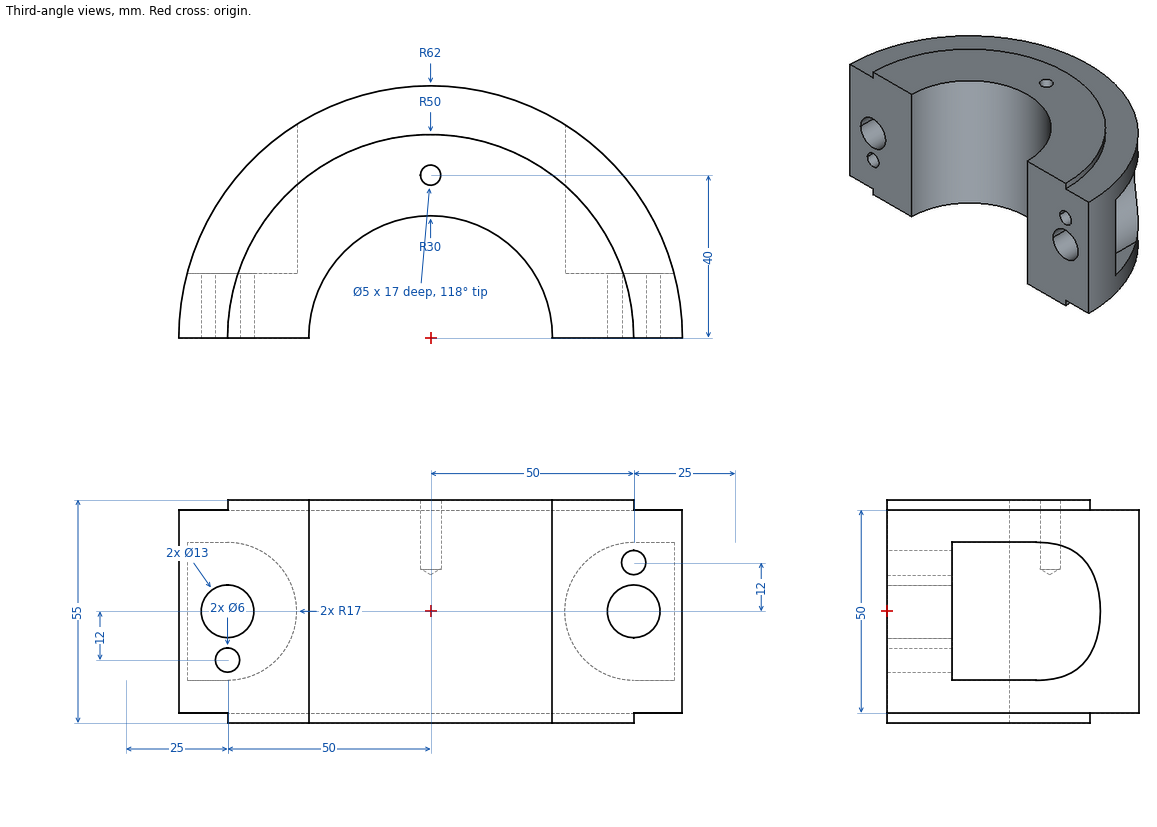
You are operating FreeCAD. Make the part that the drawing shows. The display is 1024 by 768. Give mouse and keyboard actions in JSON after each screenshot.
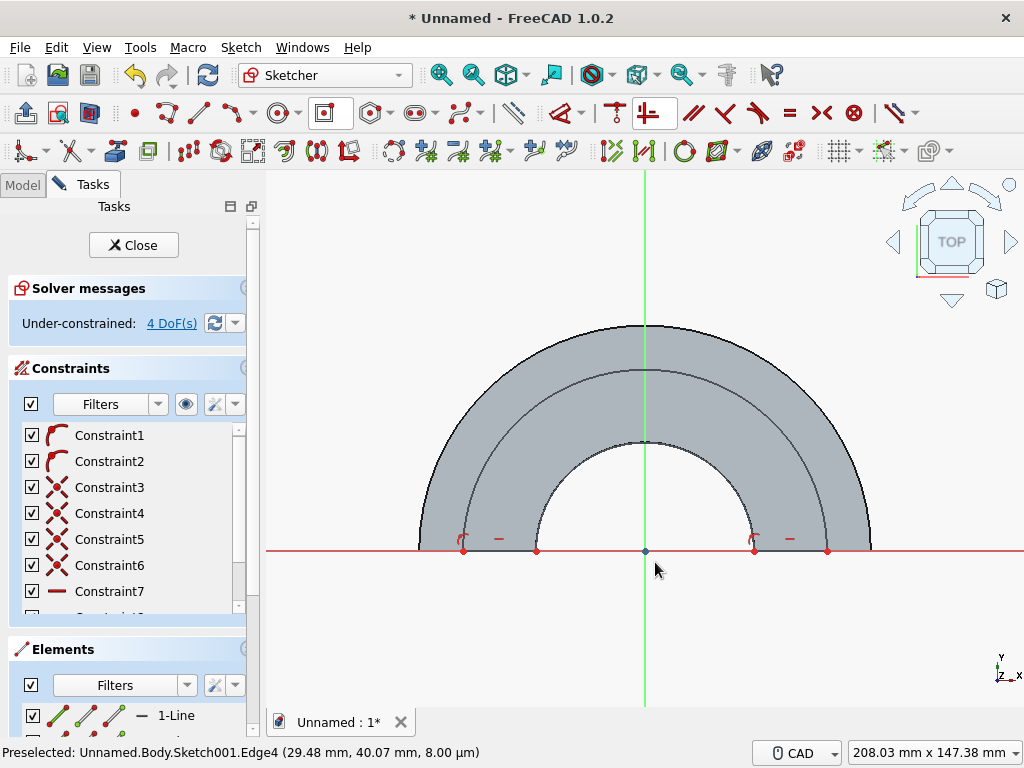
{"action": "left_click", "coordinate": [616, 114]}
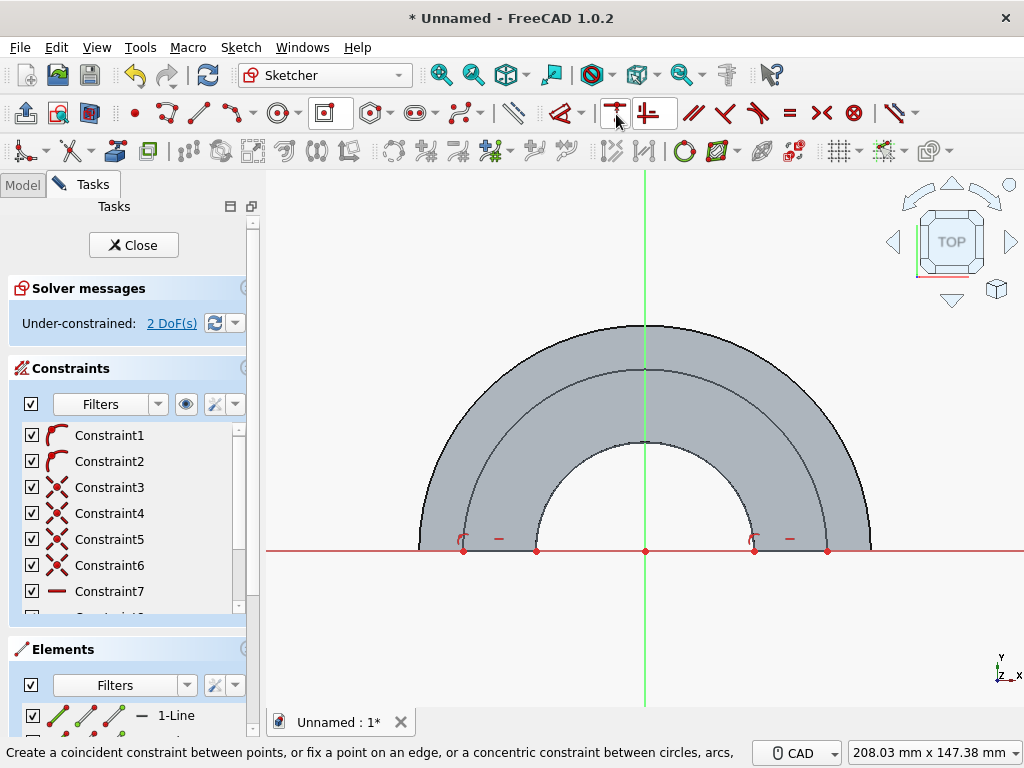
{"action": "left_click", "coordinate": [560, 114]}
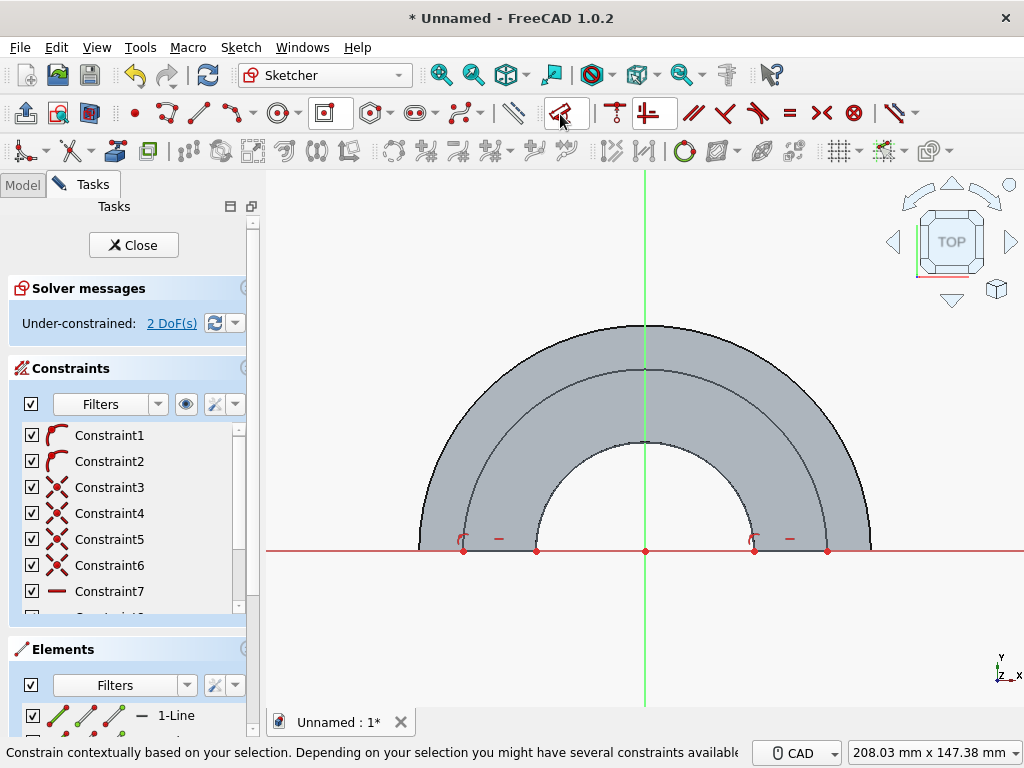
{"action": "left_click", "coordinate": [709, 463]}
{"action": "left_click", "coordinate": [728, 437]}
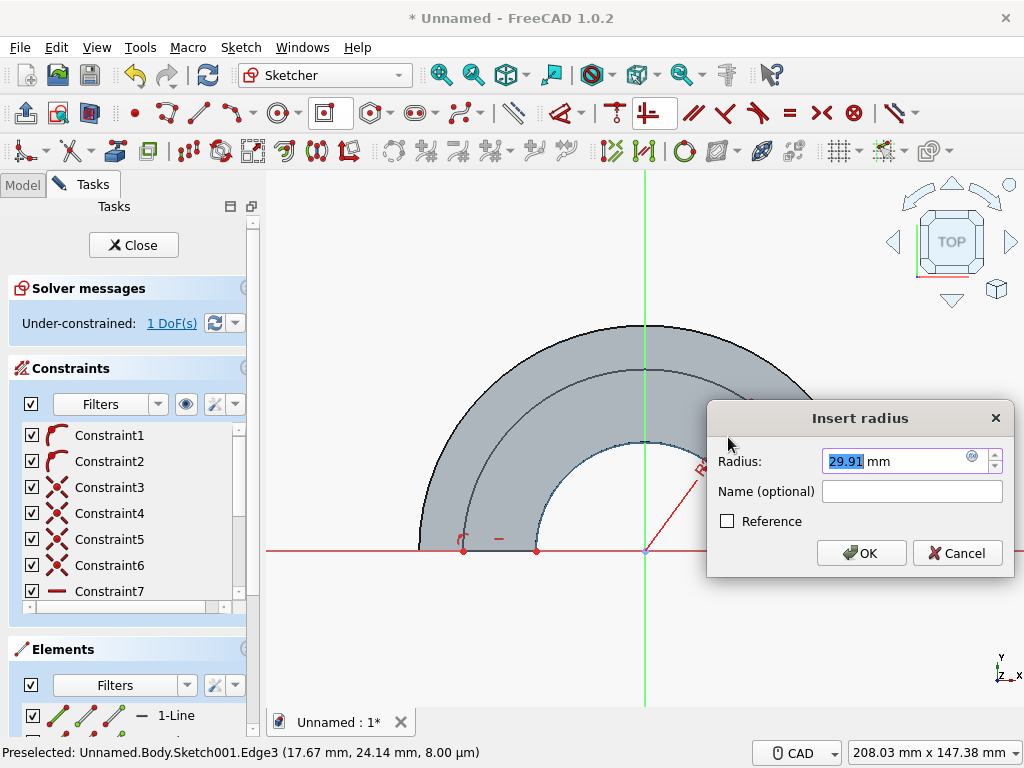
{"action": "type", "text": "30"}
{"action": "key", "text": "Return"}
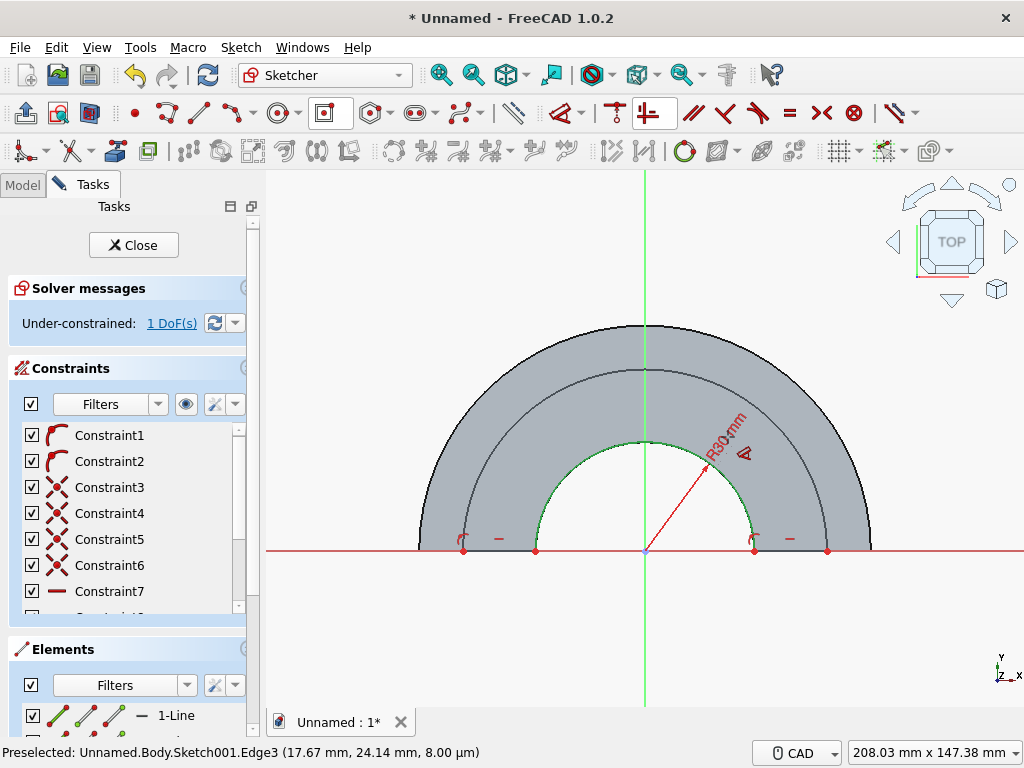
{"action": "left_click", "coordinate": [752, 404]}
{"action": "left_click", "coordinate": [771, 378]}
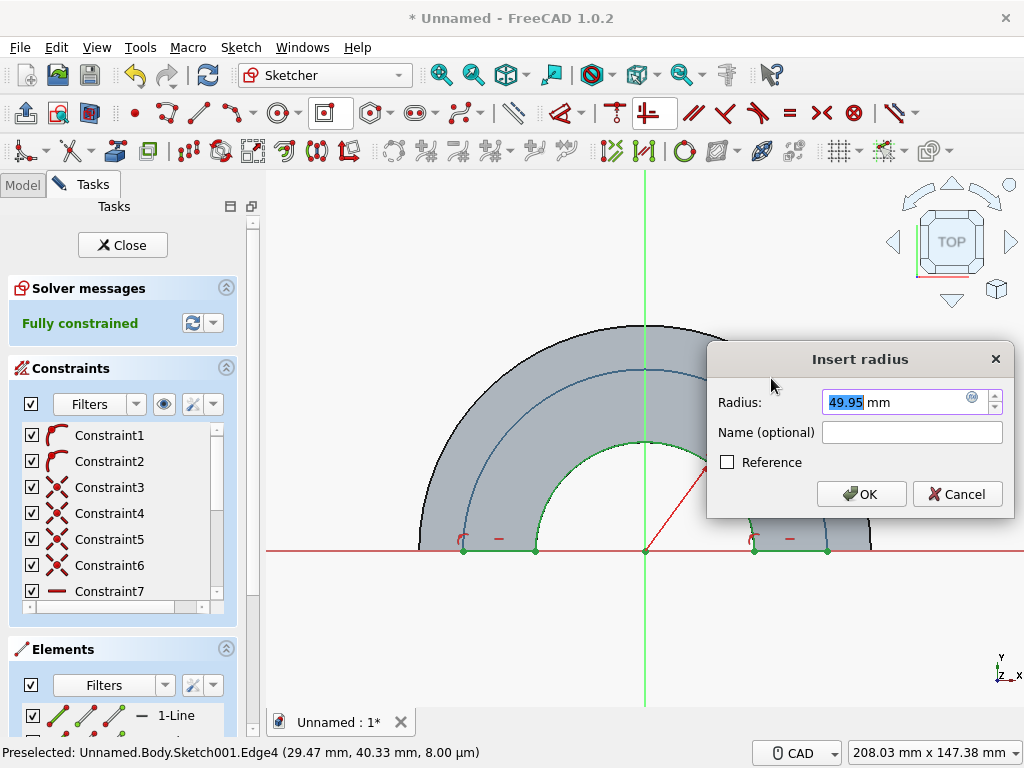
{"action": "type", "text": "50"}
{"action": "key", "text": "Return"}
{"action": "key", "text": "Escape"}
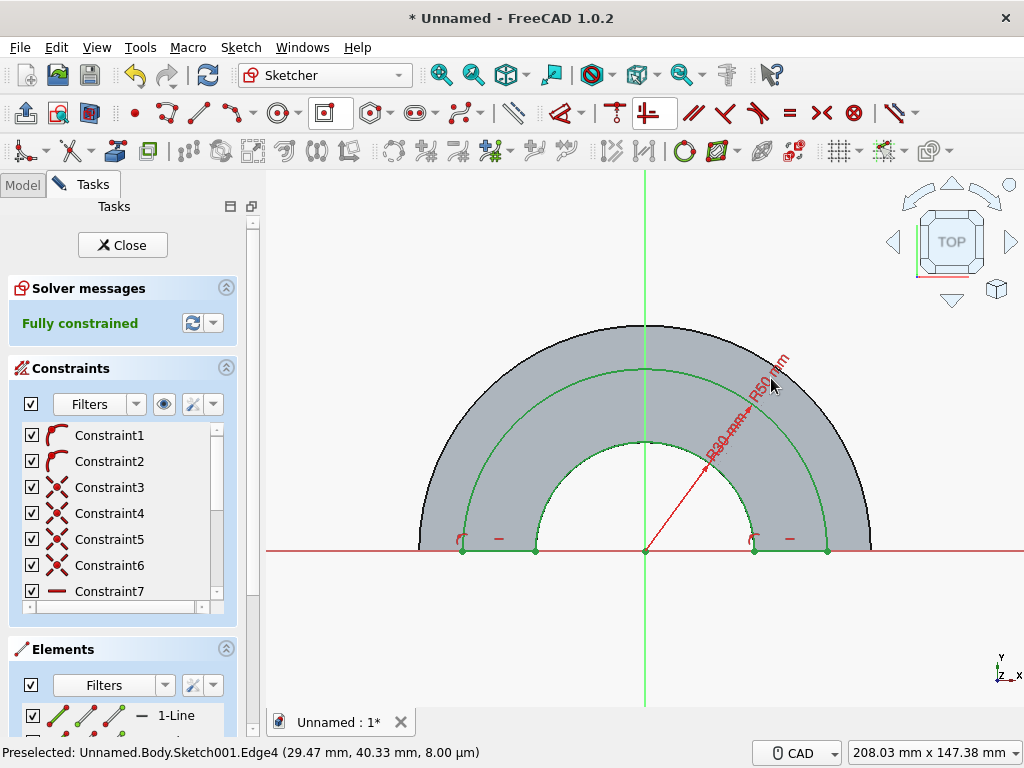
{"action": "left_click", "coordinate": [123, 245]}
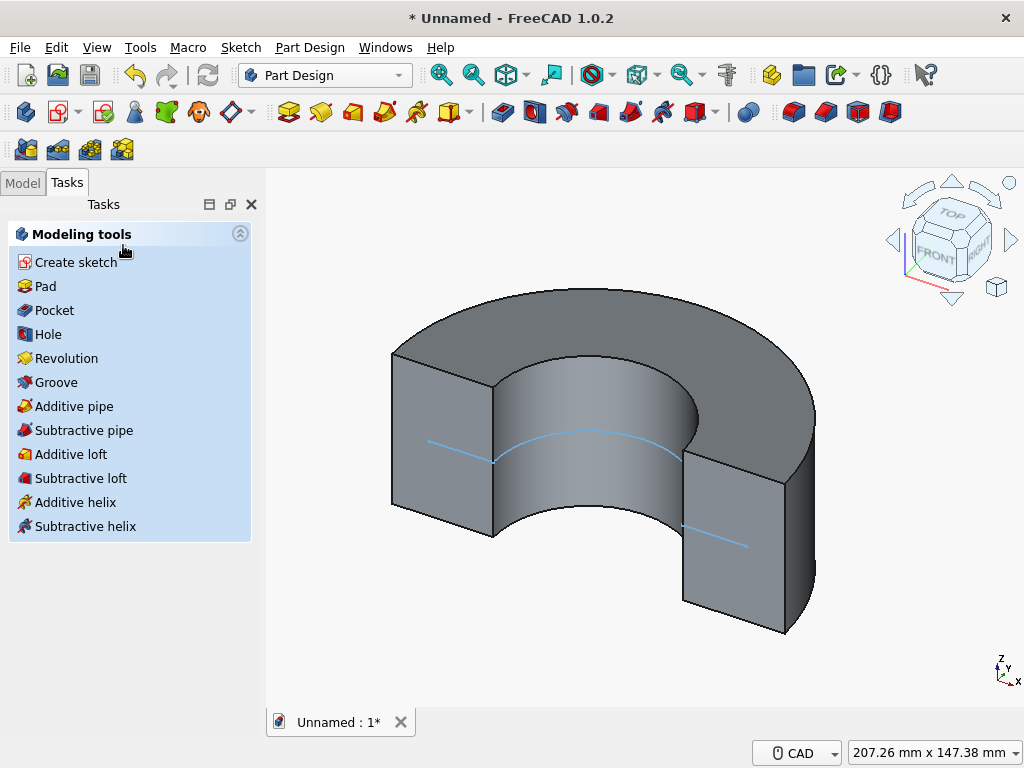
{"action": "left_click", "coordinate": [290, 112]}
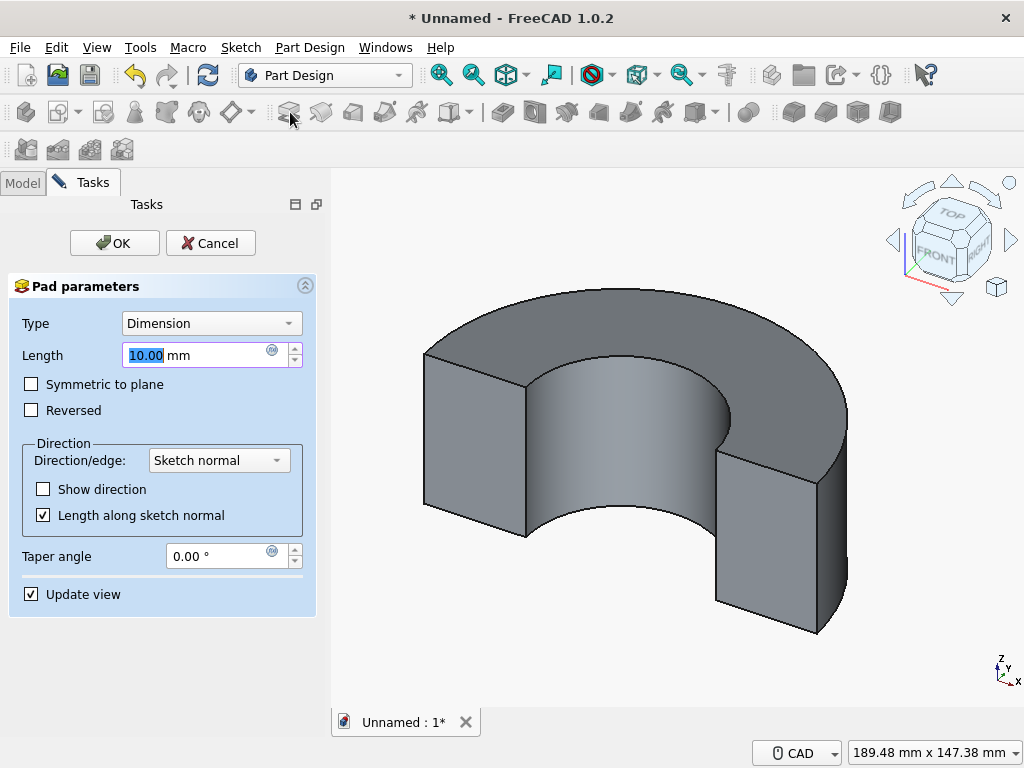
{"action": "type", "text": "55"}
{"action": "key", "text": "Tab"}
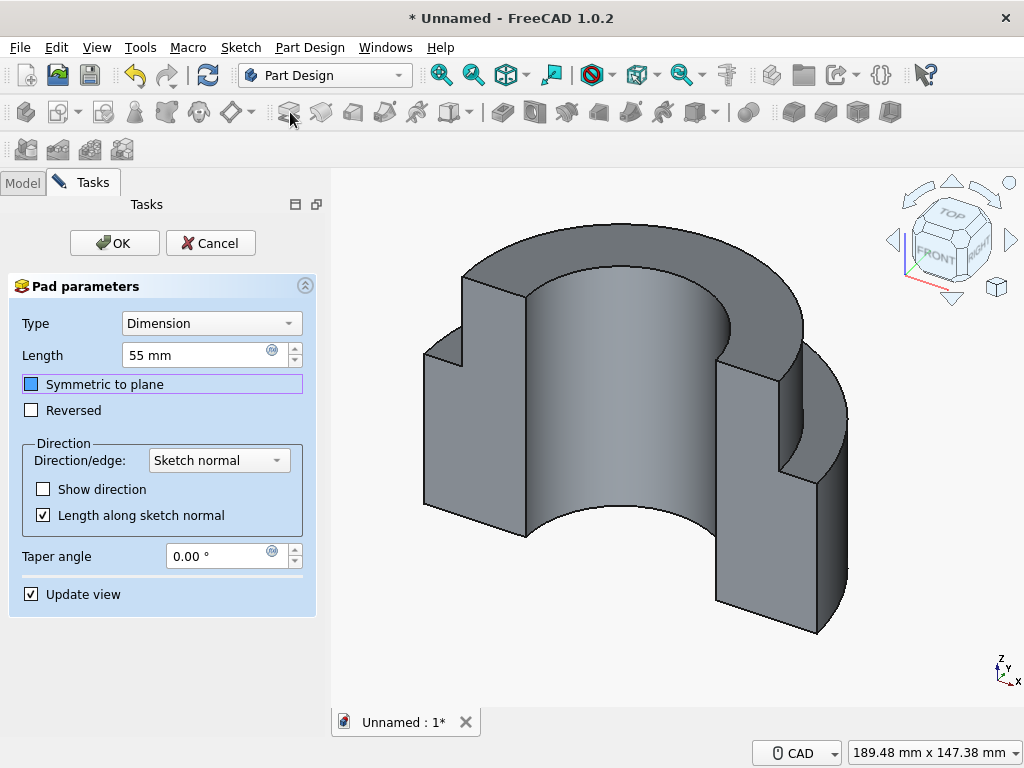
{"action": "left_click", "coordinate": [30, 384]}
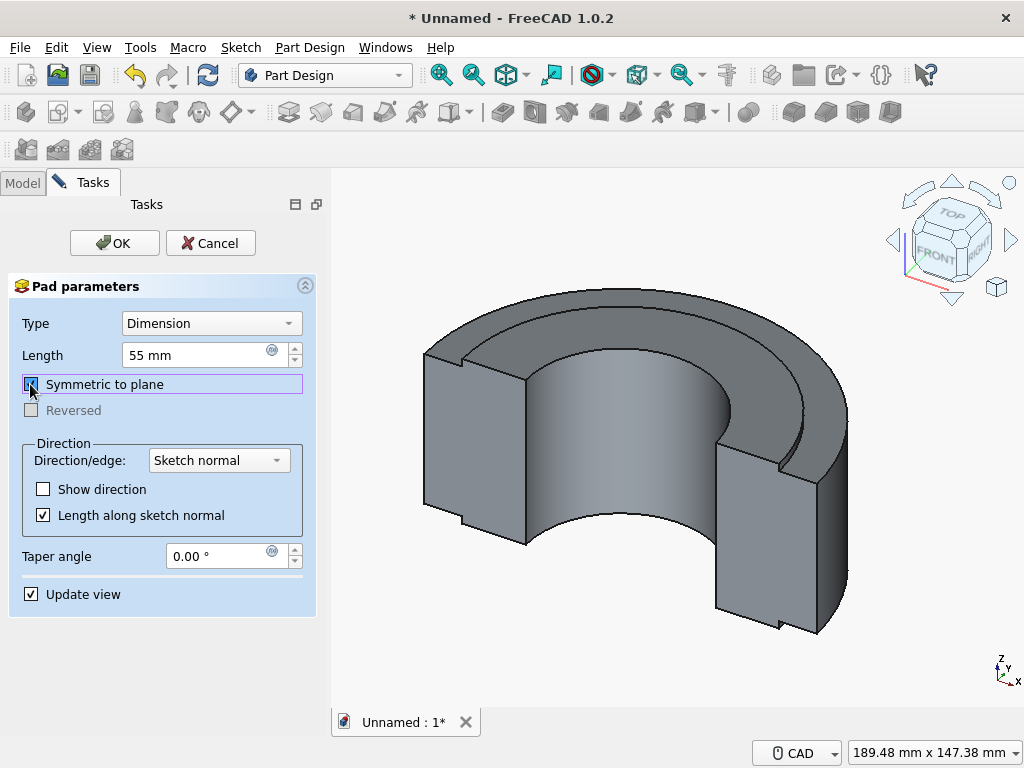
{"action": "left_click", "coordinate": [115, 243]}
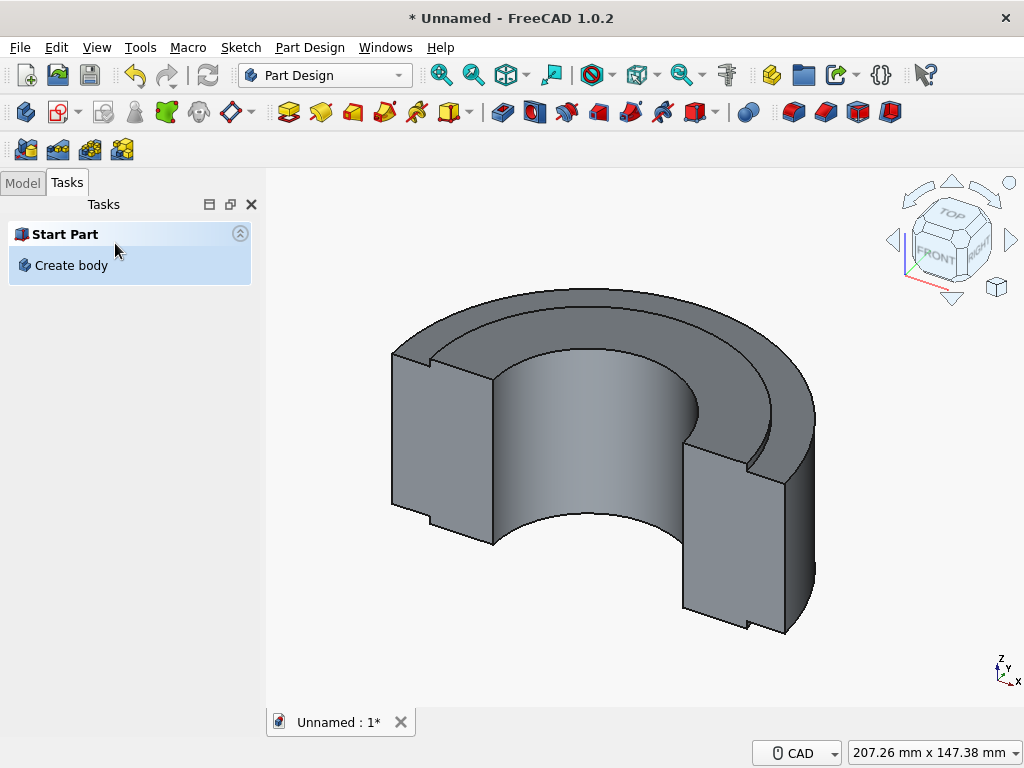
{"action": "left_click", "coordinate": [23, 182]}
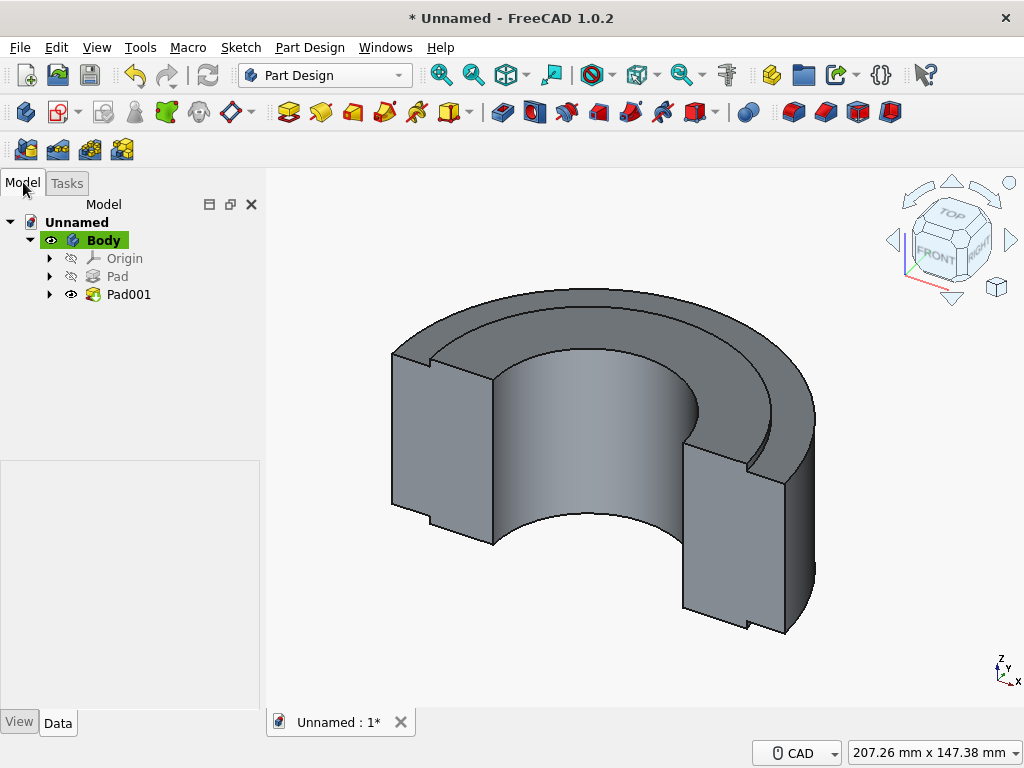
{"action": "left_click", "coordinate": [50, 258]}